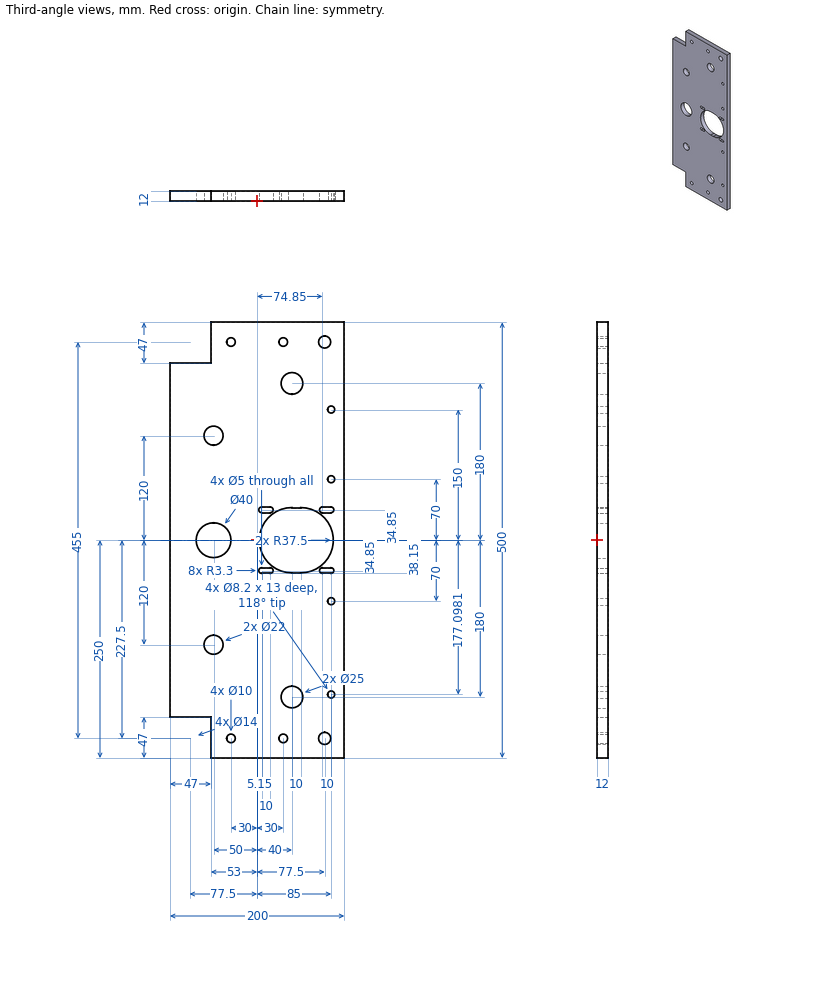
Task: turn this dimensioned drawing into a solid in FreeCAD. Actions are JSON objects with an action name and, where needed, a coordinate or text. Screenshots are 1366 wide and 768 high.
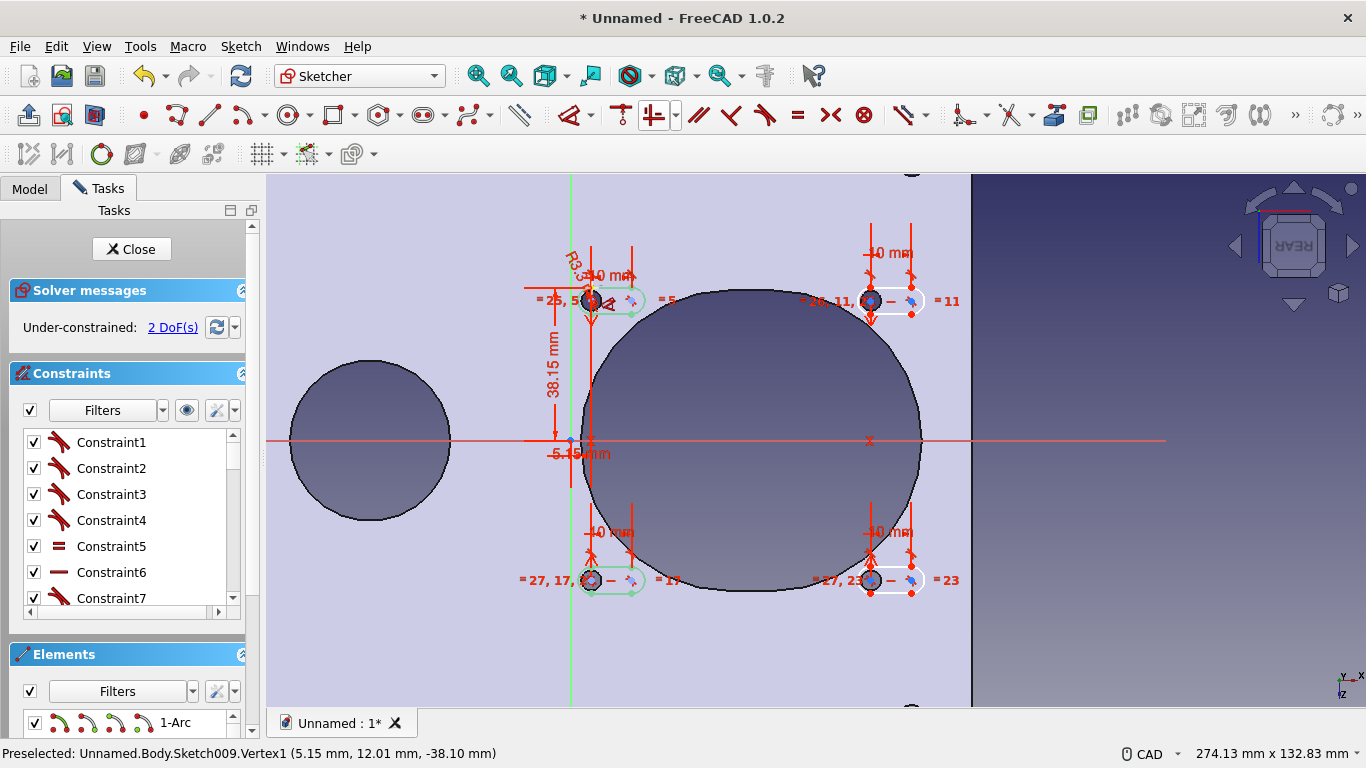
{"action": "left_click", "coordinate": [871, 288]}
{"action": "left_click", "coordinate": [721, 254]}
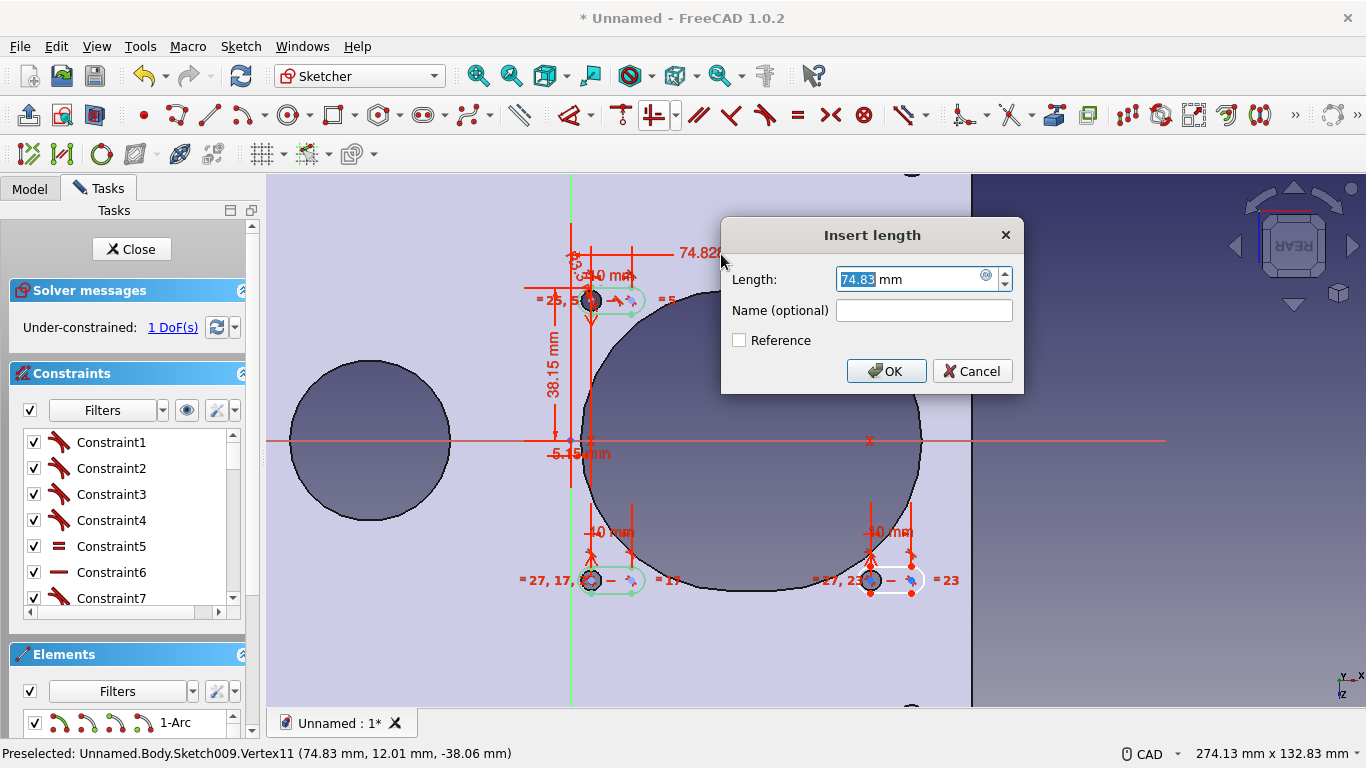
{"action": "type", "text": "74.85"}
{"action": "key", "text": "Return"}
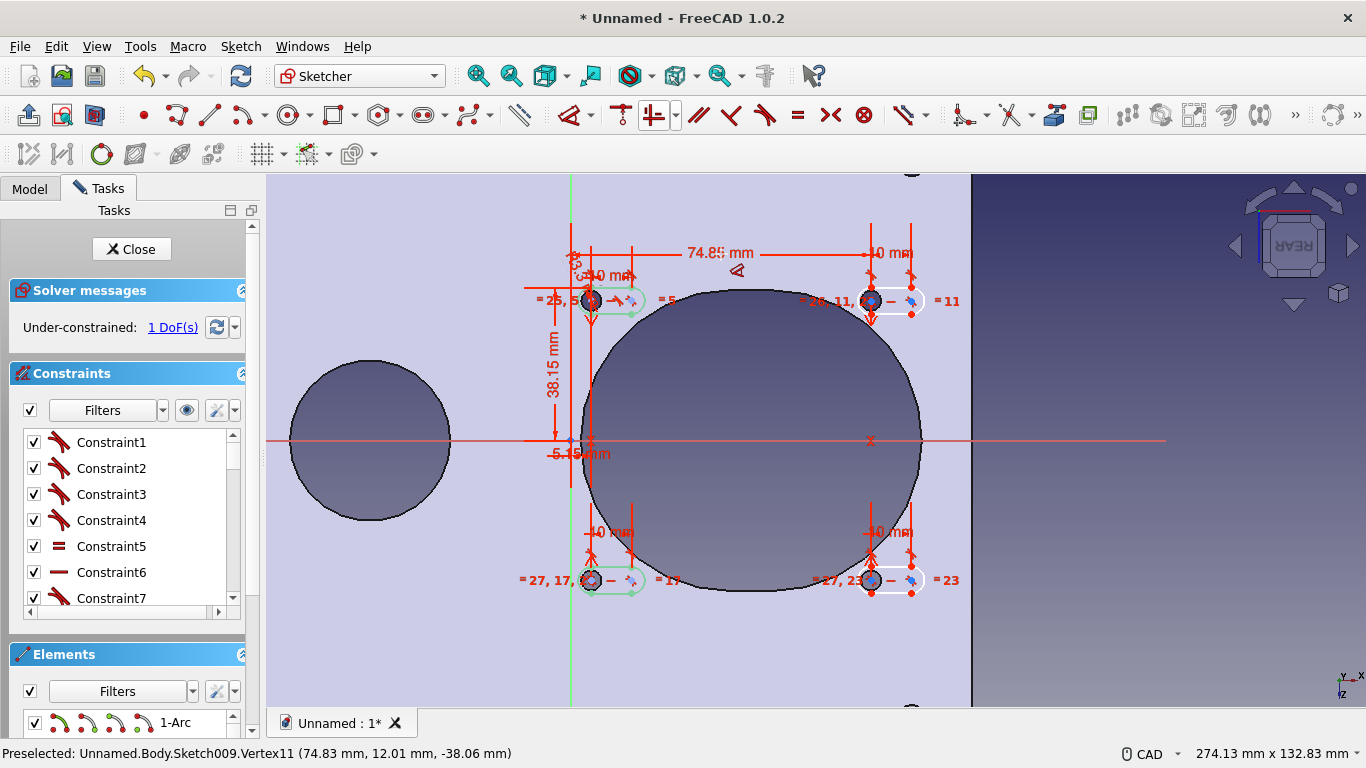
{"action": "left_click", "coordinate": [871, 288]}
{"action": "left_click", "coordinate": [537, 329]}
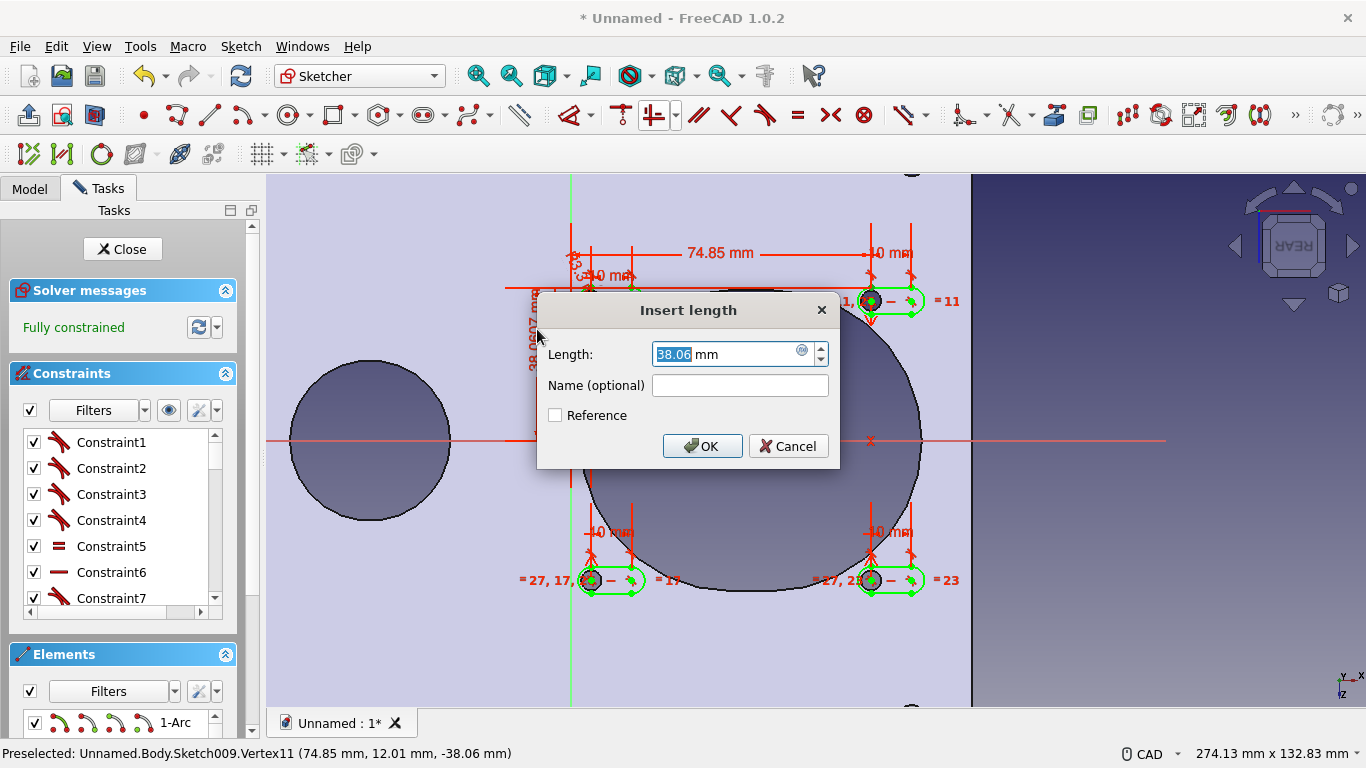
{"action": "type", "text": "38.15"}
{"action": "key", "text": "Return"}
{"action": "key", "text": "Escape"}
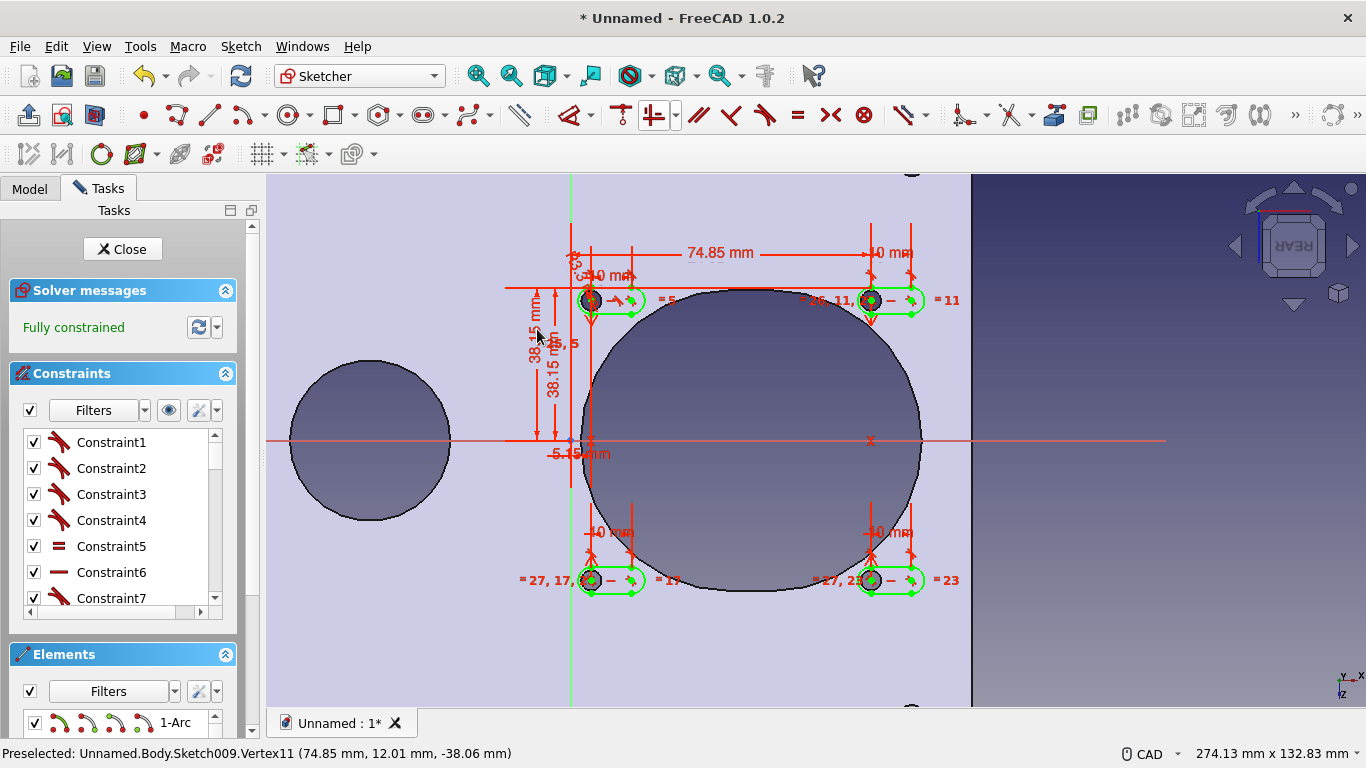
{"action": "left_click", "coordinate": [123, 249]}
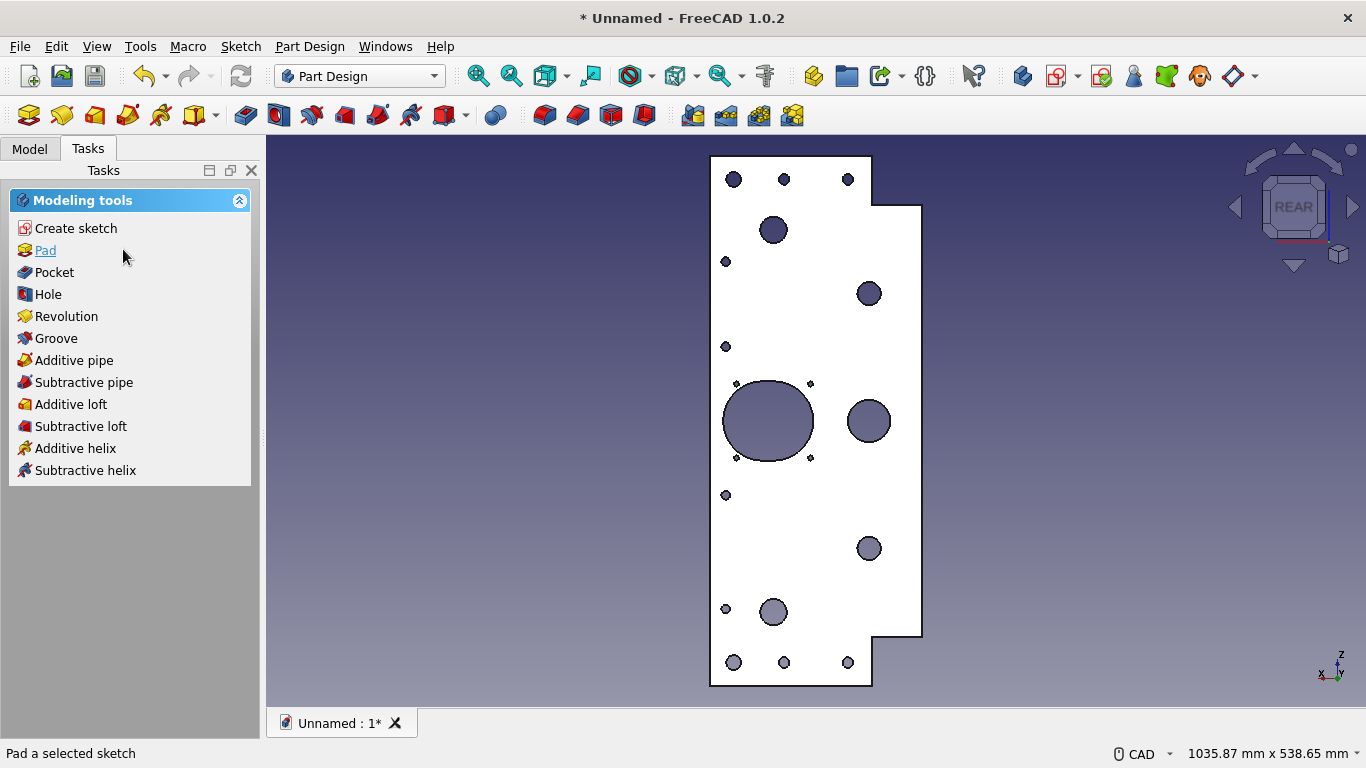
{"action": "left_click", "coordinate": [246, 116]}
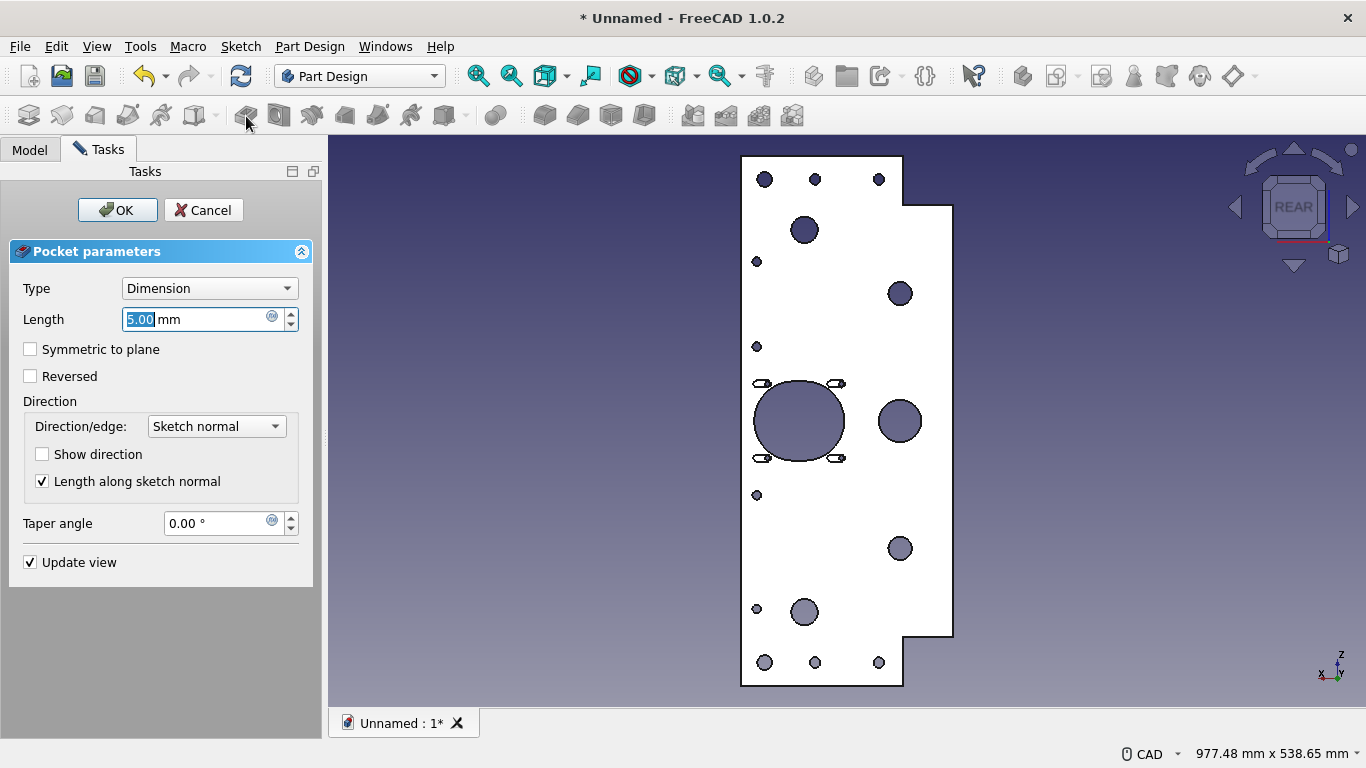
{"action": "left_click", "coordinate": [210, 288]}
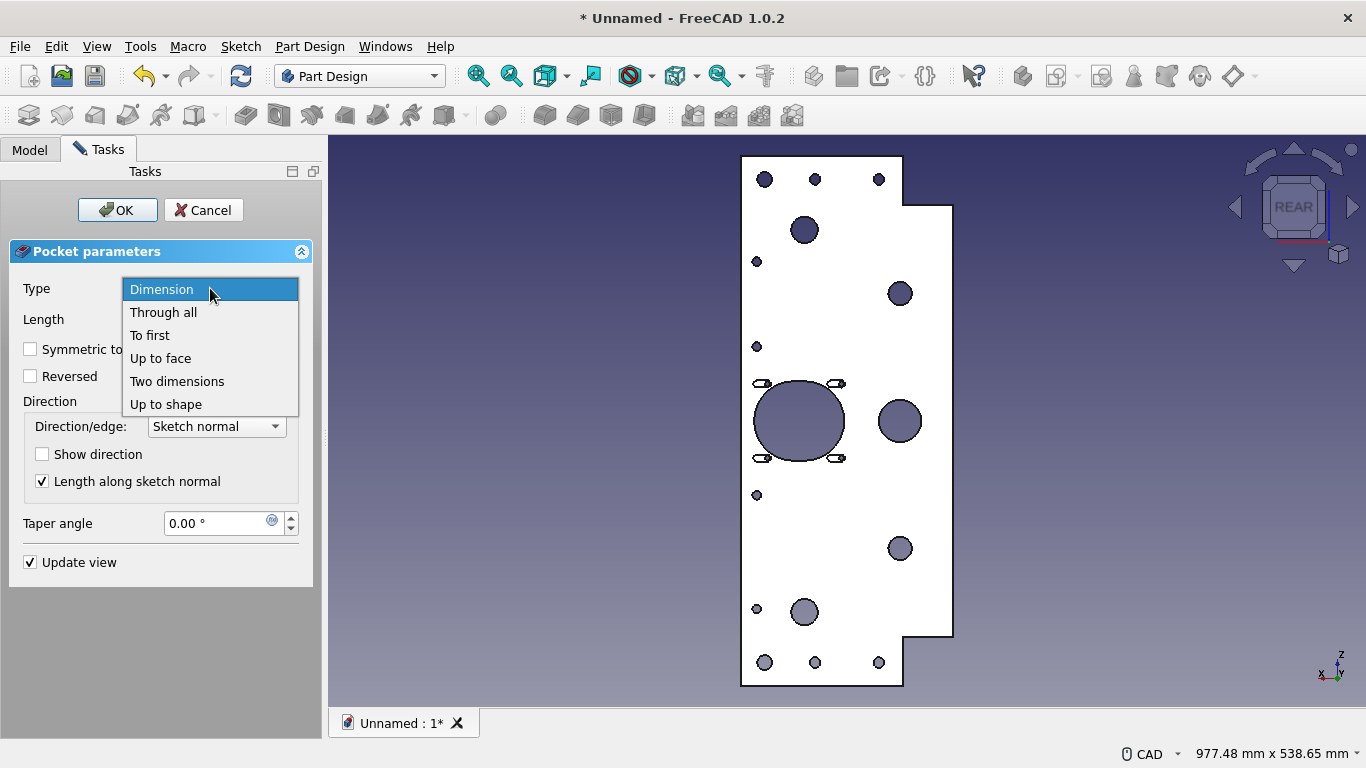
{"action": "left_click", "coordinate": [208, 312]}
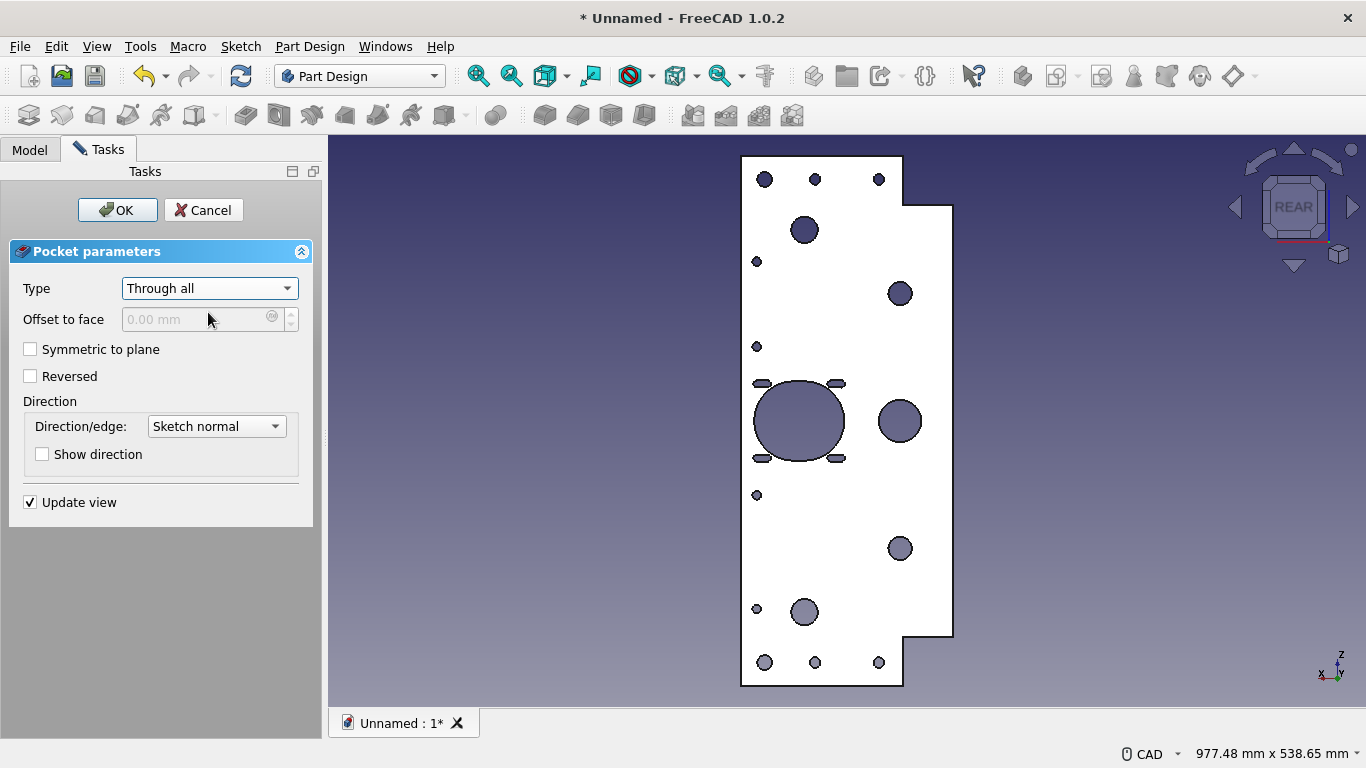
{"action": "left_click", "coordinate": [118, 210]}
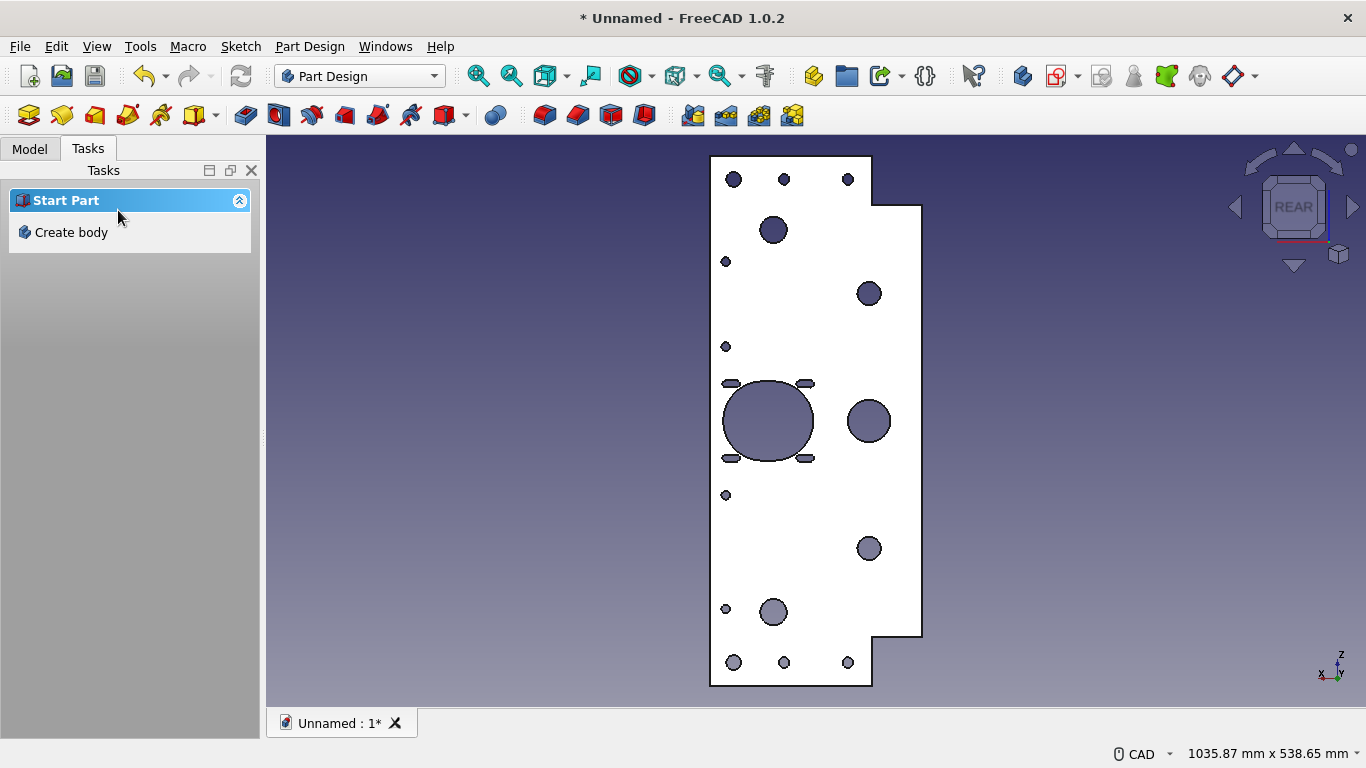
{"action": "key", "text": "0"}